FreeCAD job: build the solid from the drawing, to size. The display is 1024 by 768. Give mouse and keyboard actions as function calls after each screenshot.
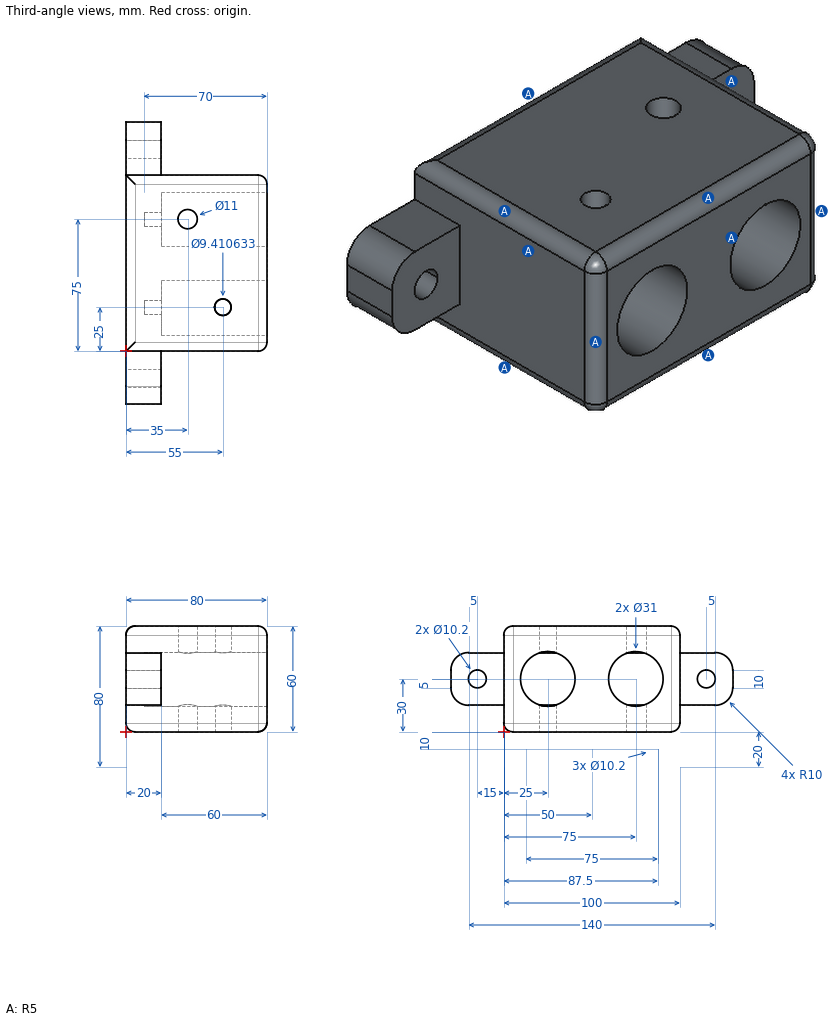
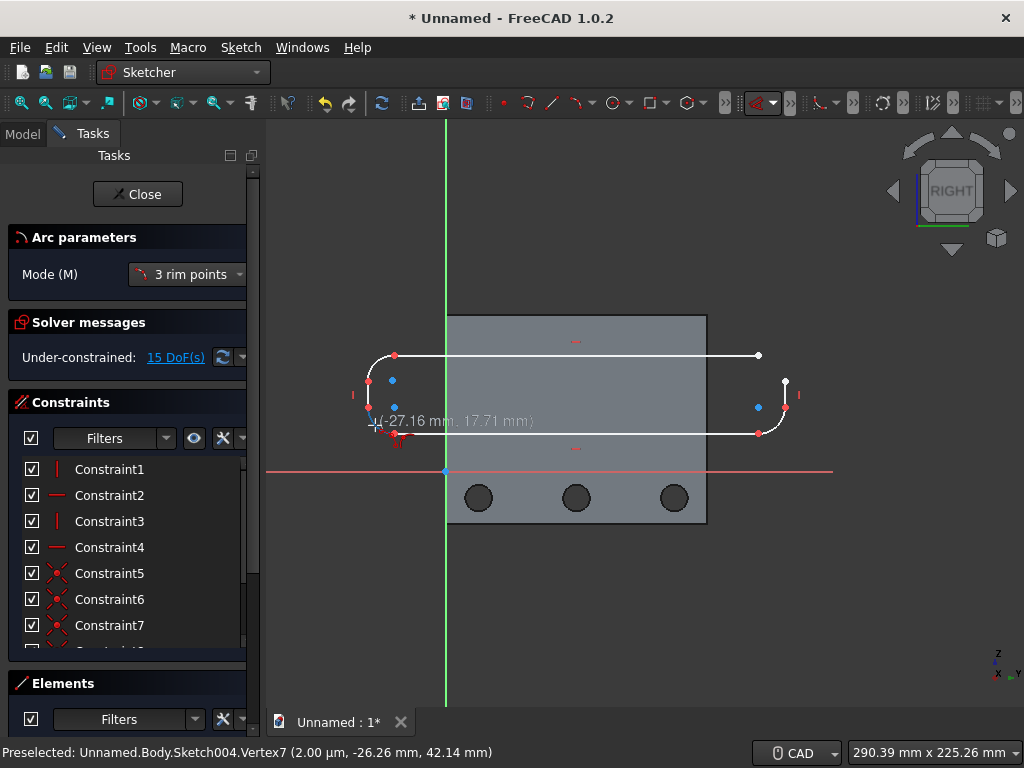
click(759, 356)
click(785, 382)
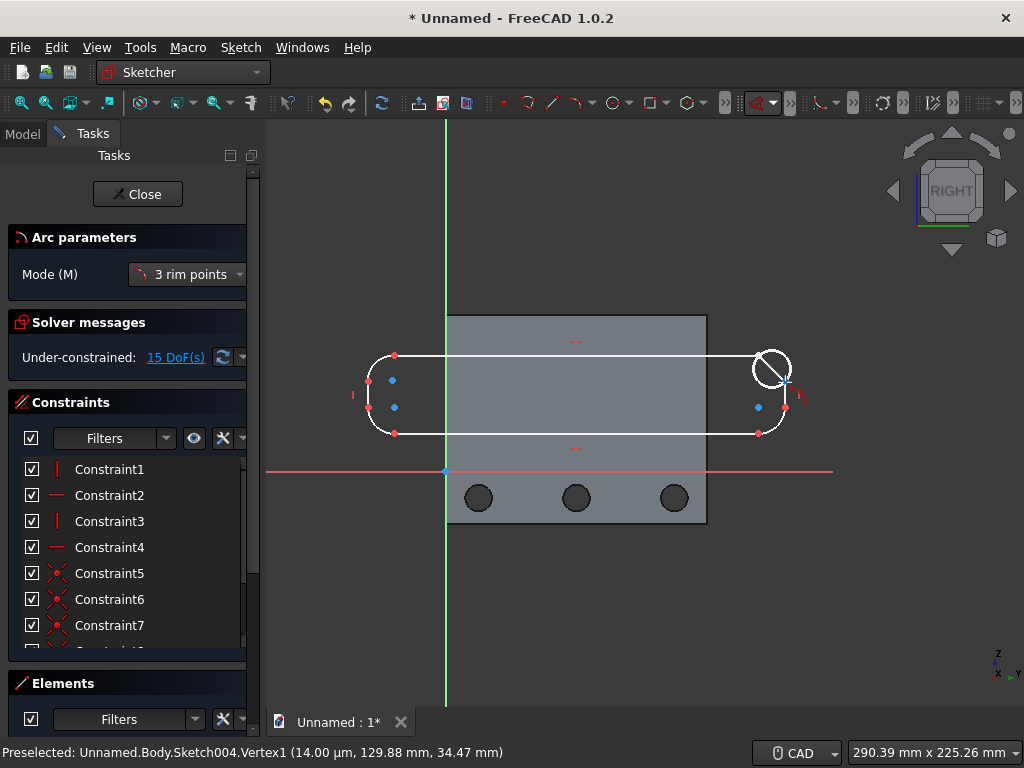
scroll(778, 362, up, 4)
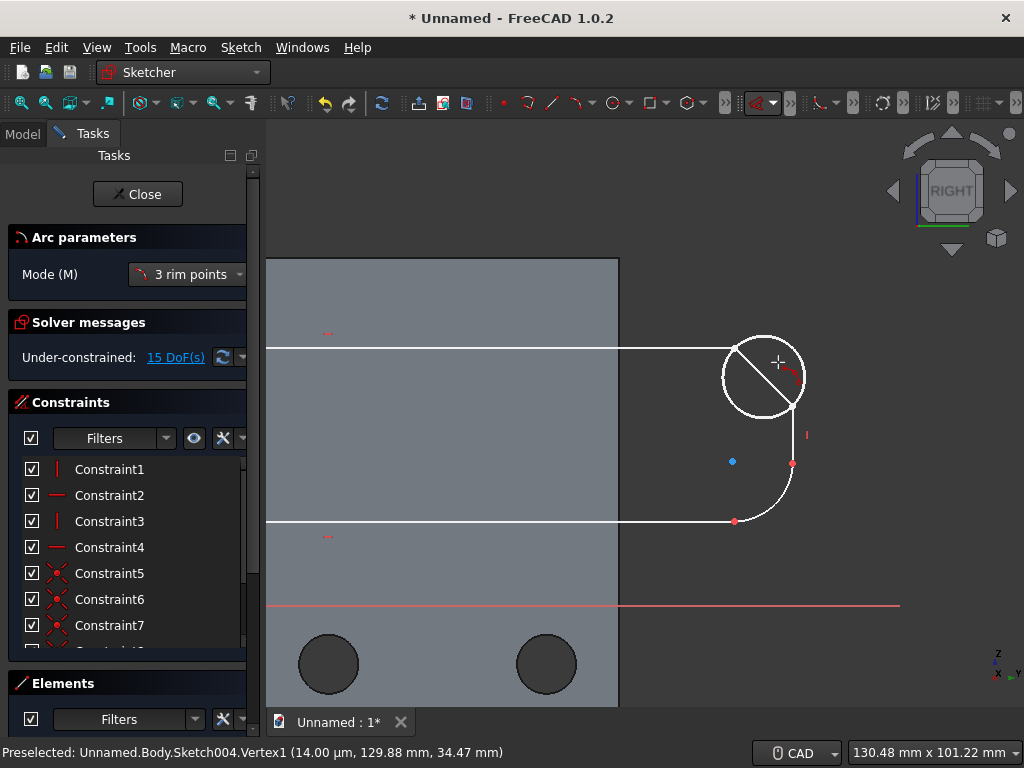
click(776, 362)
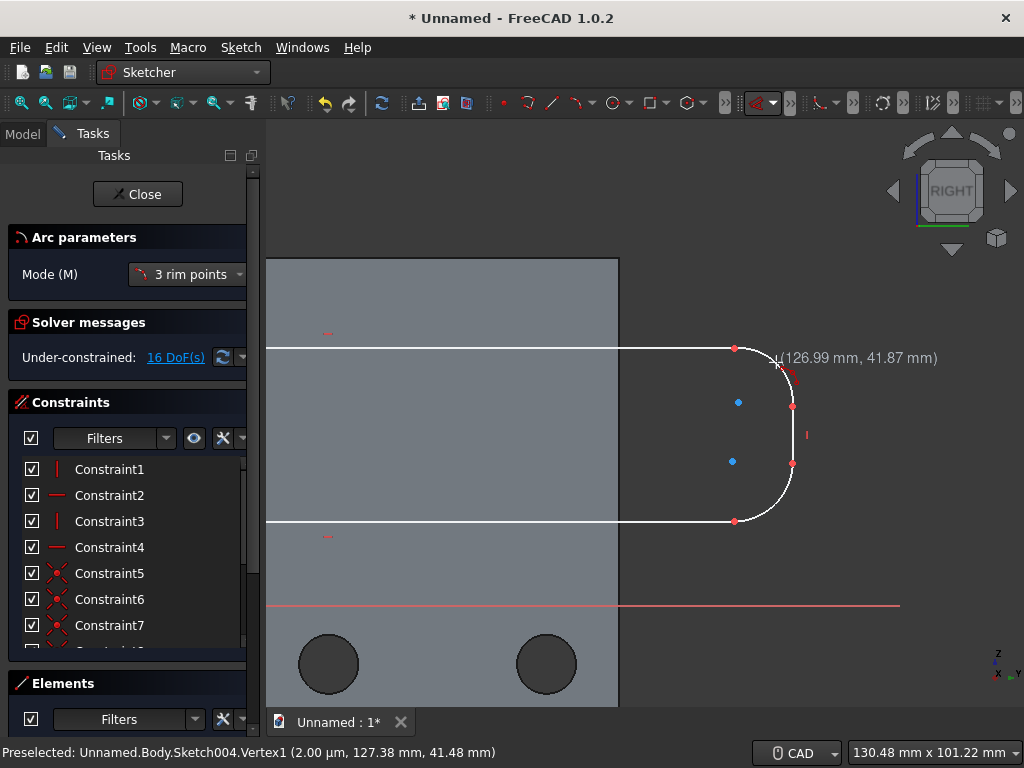
key(g)
key(c)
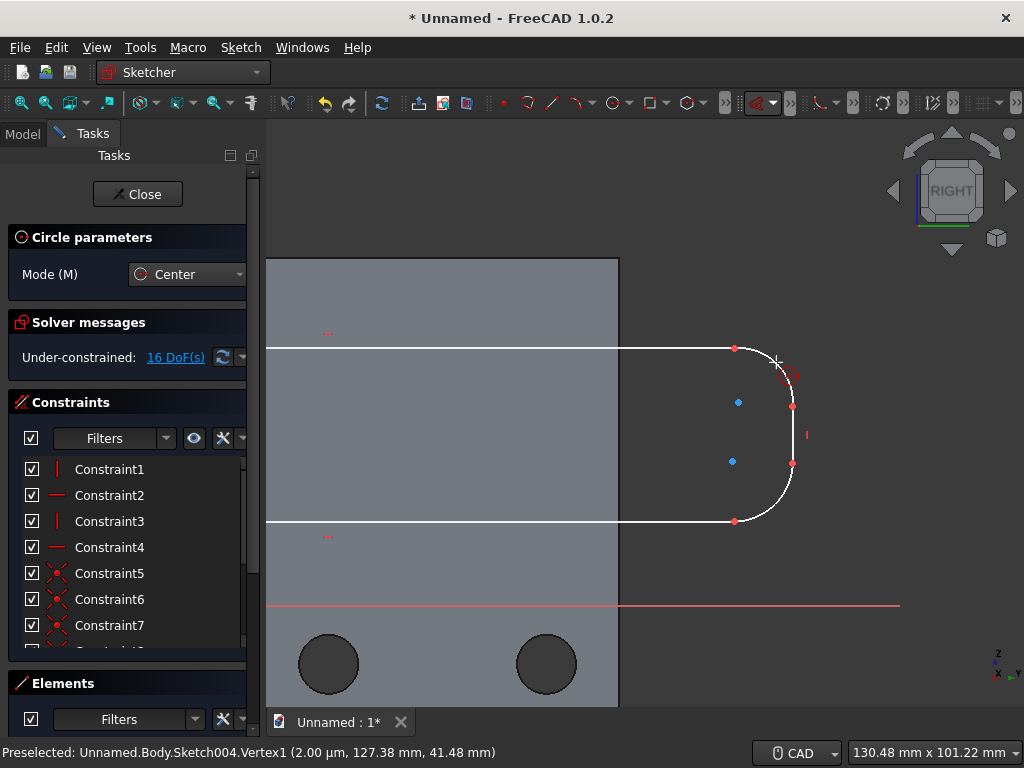
scroll(779, 362, down, 4)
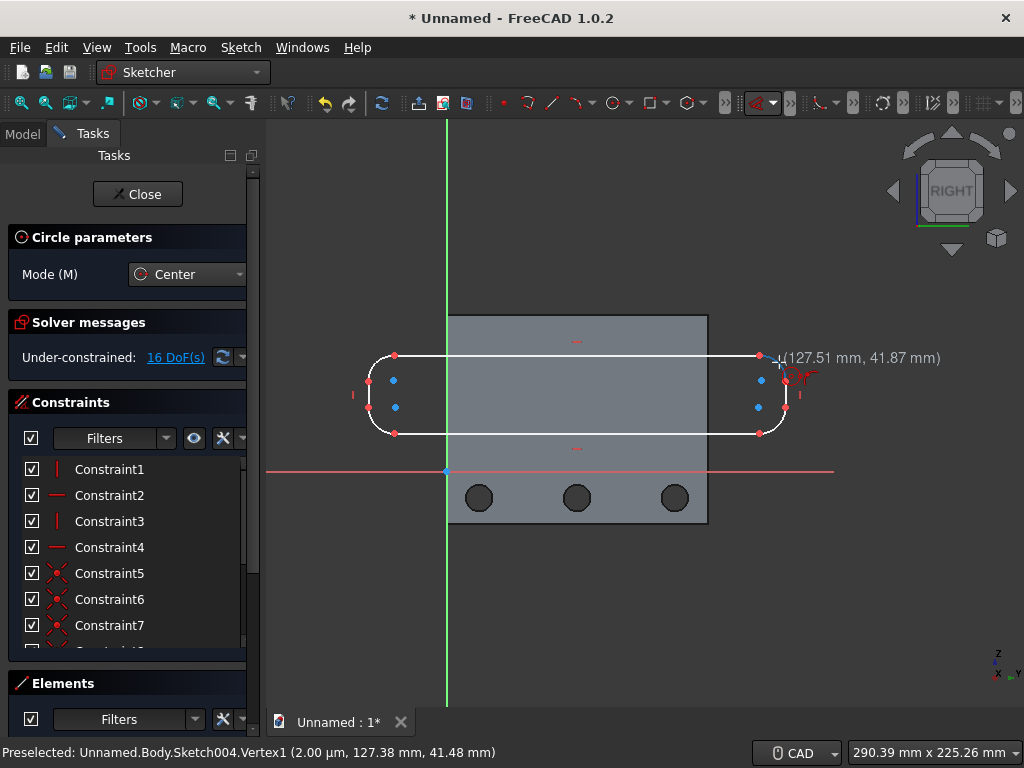
scroll(407, 394, up, 3)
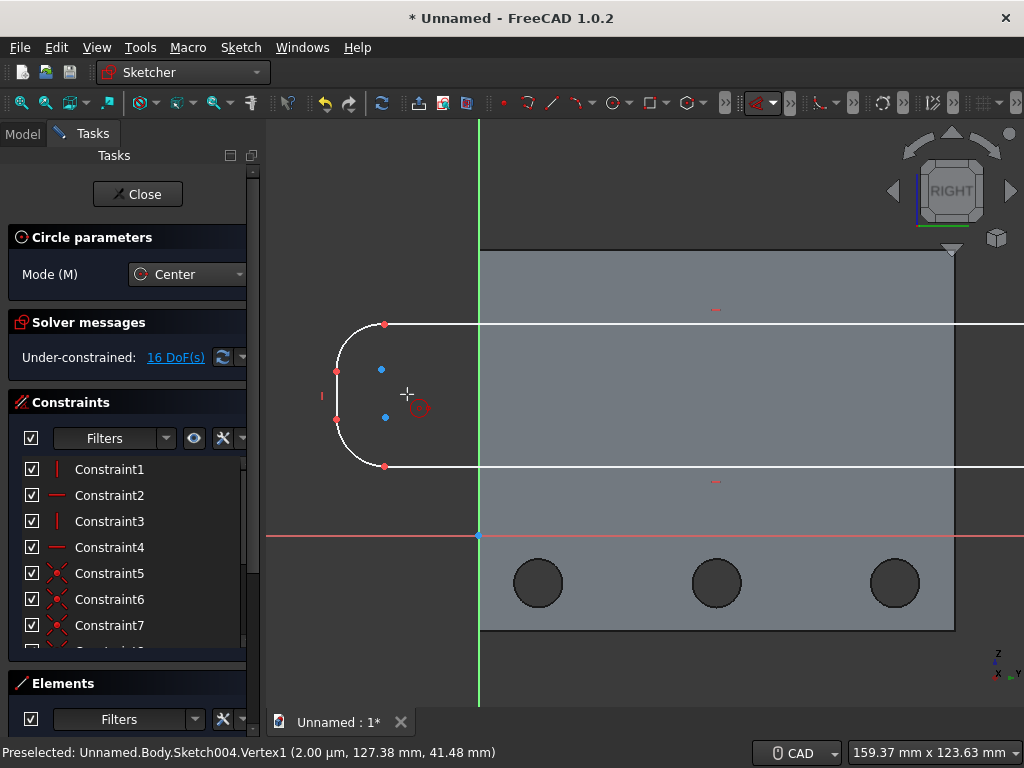
click(408, 393)
move(425, 376)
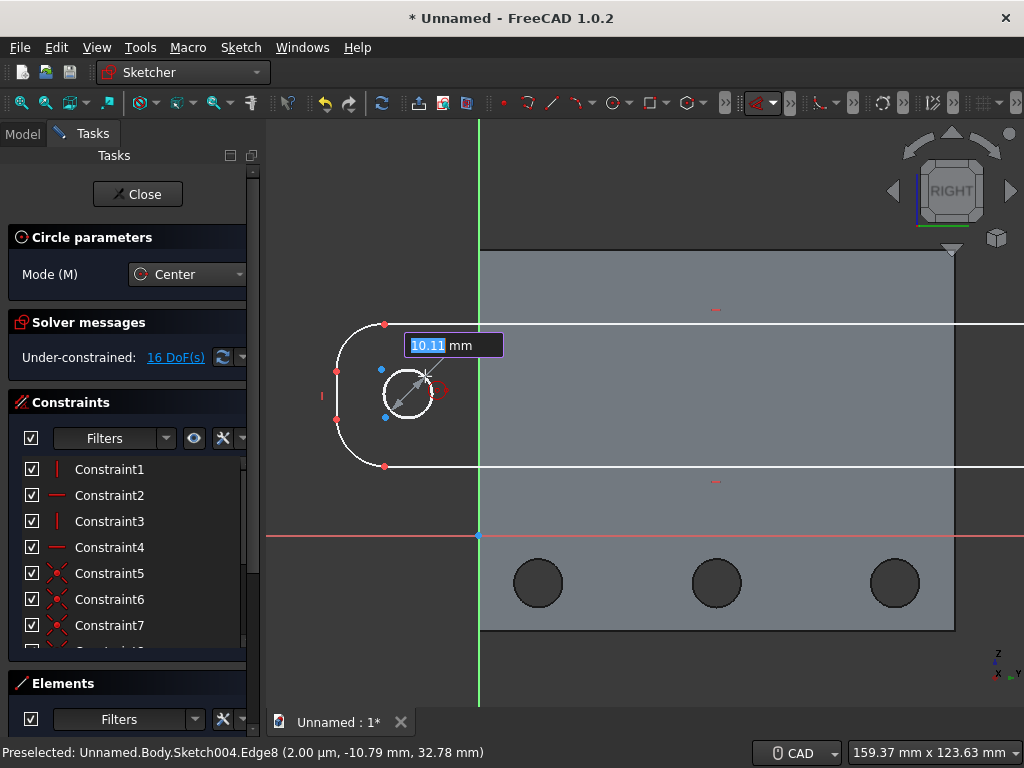
text(10.2)
key(Return)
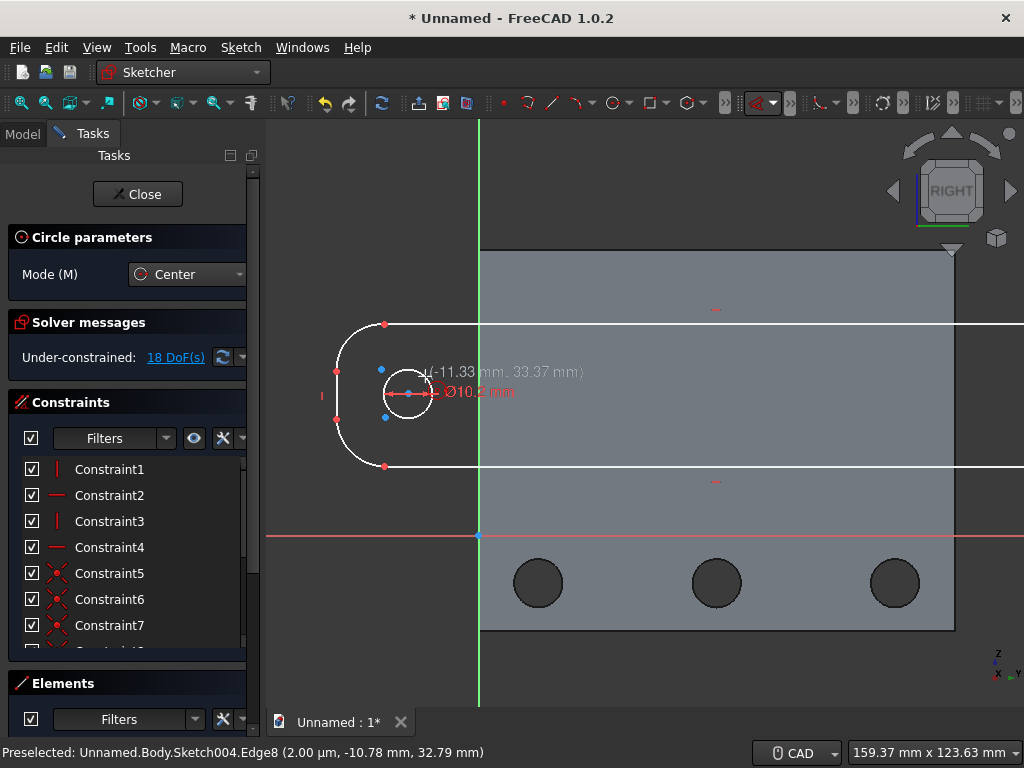
scroll(406, 394, down, 3)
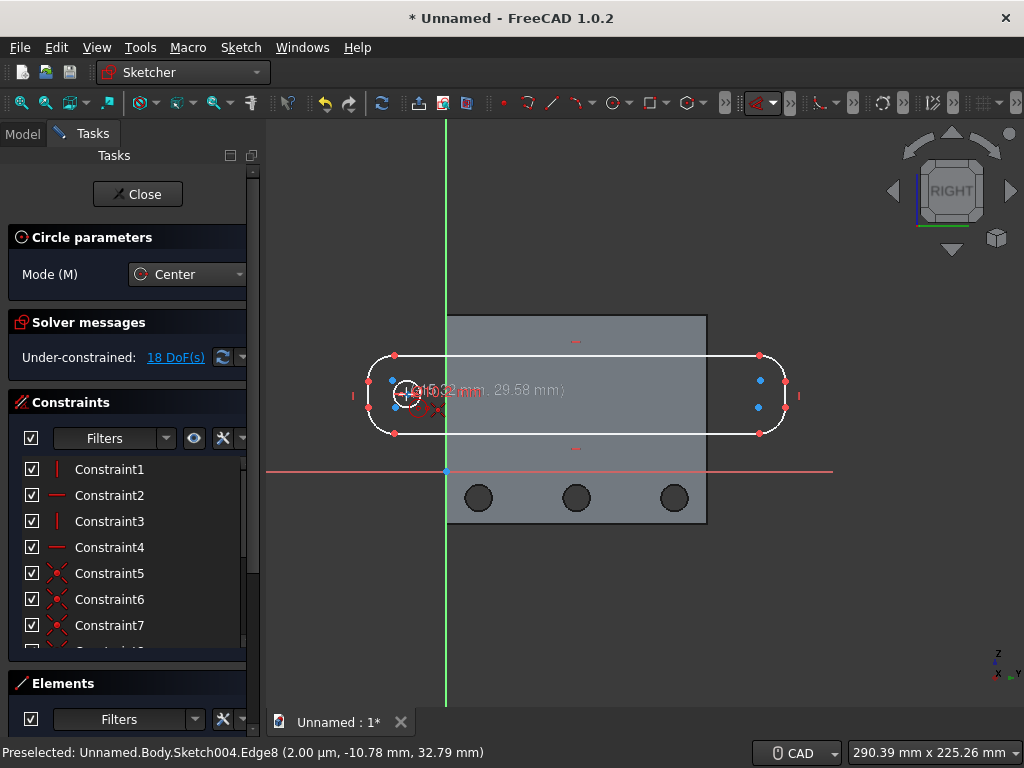
scroll(746, 394, up, 3)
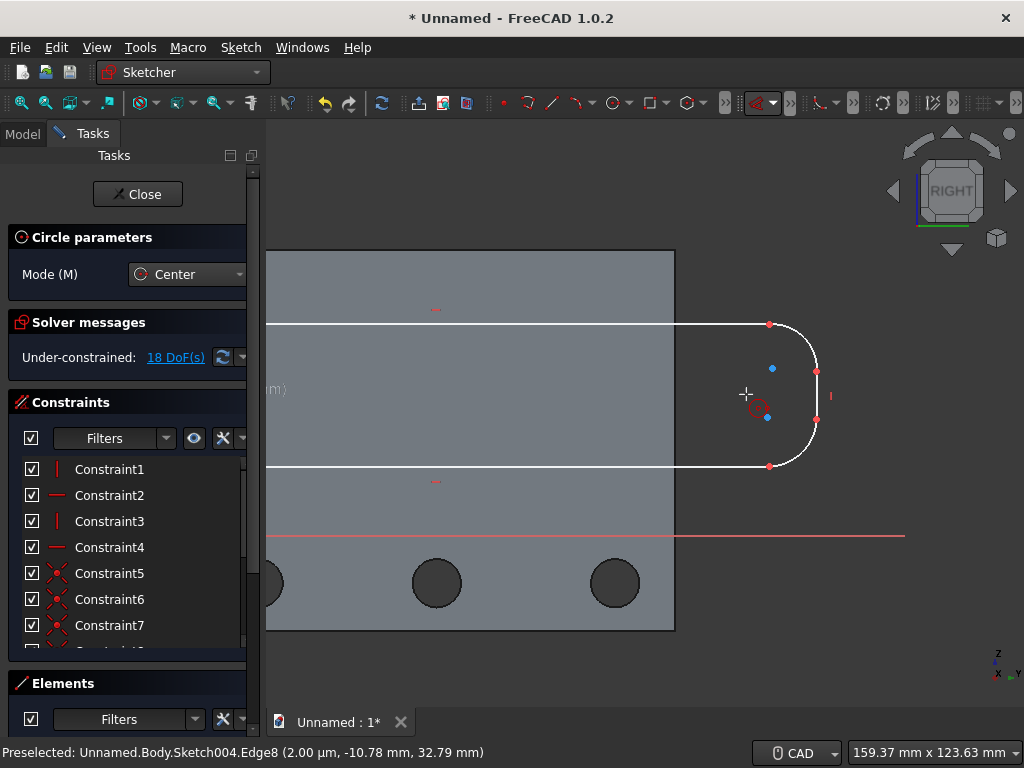
click(746, 393)
move(729, 376)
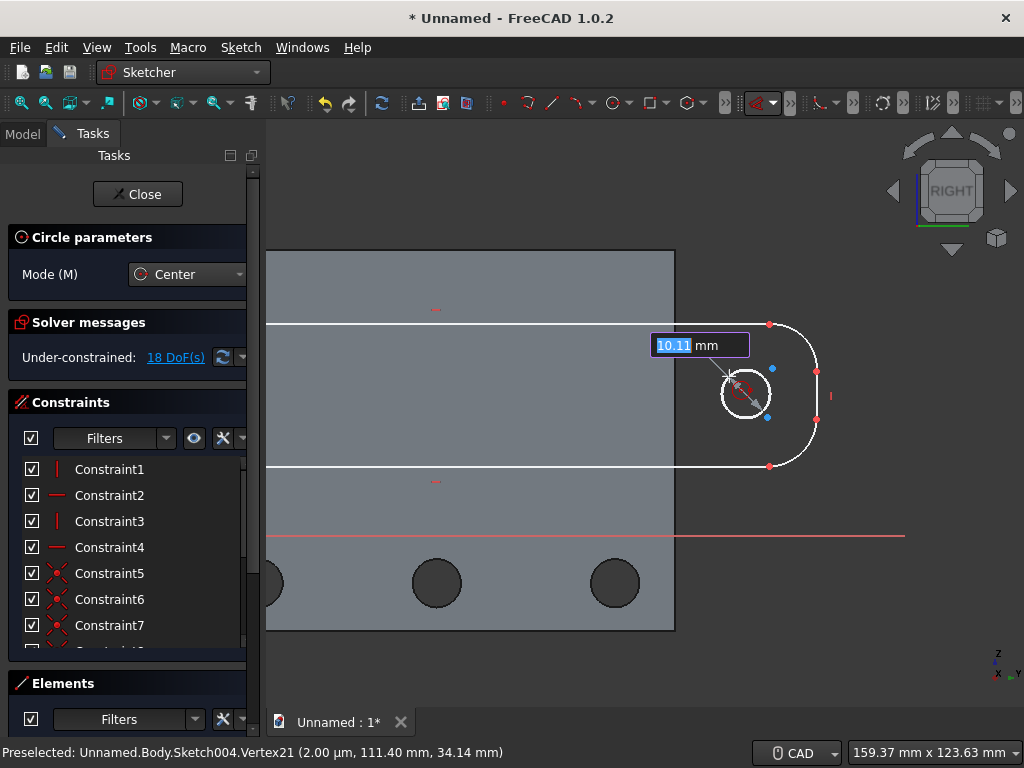
text(10.2)
key(Return)
key(Escape)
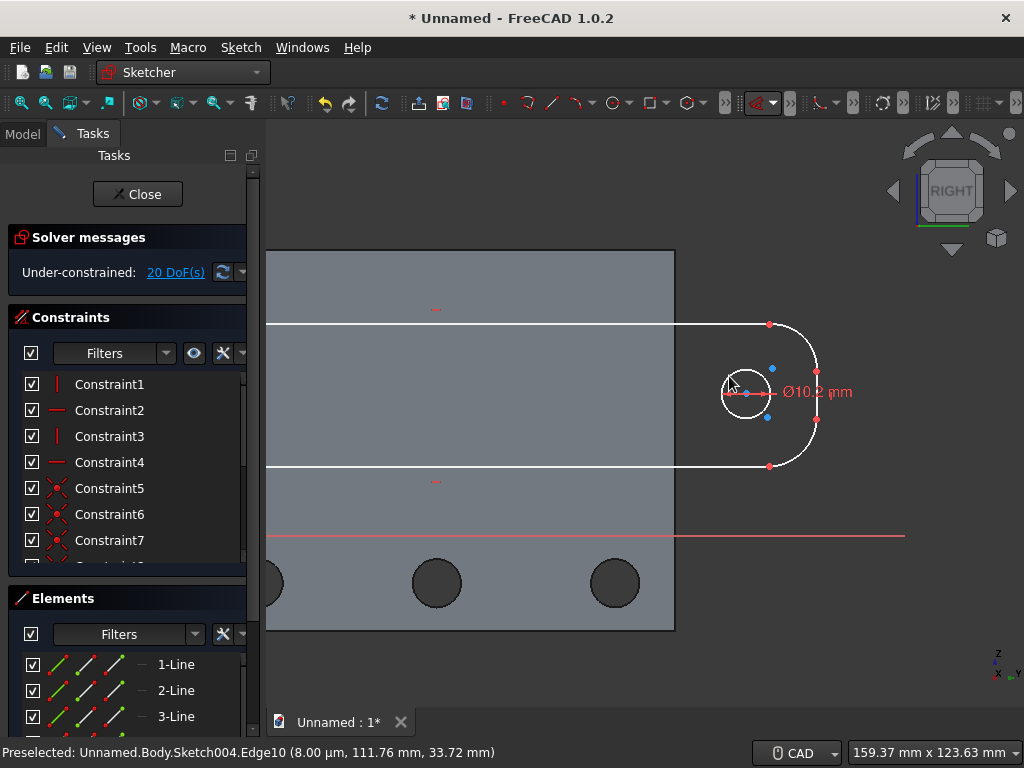
click(817, 386)